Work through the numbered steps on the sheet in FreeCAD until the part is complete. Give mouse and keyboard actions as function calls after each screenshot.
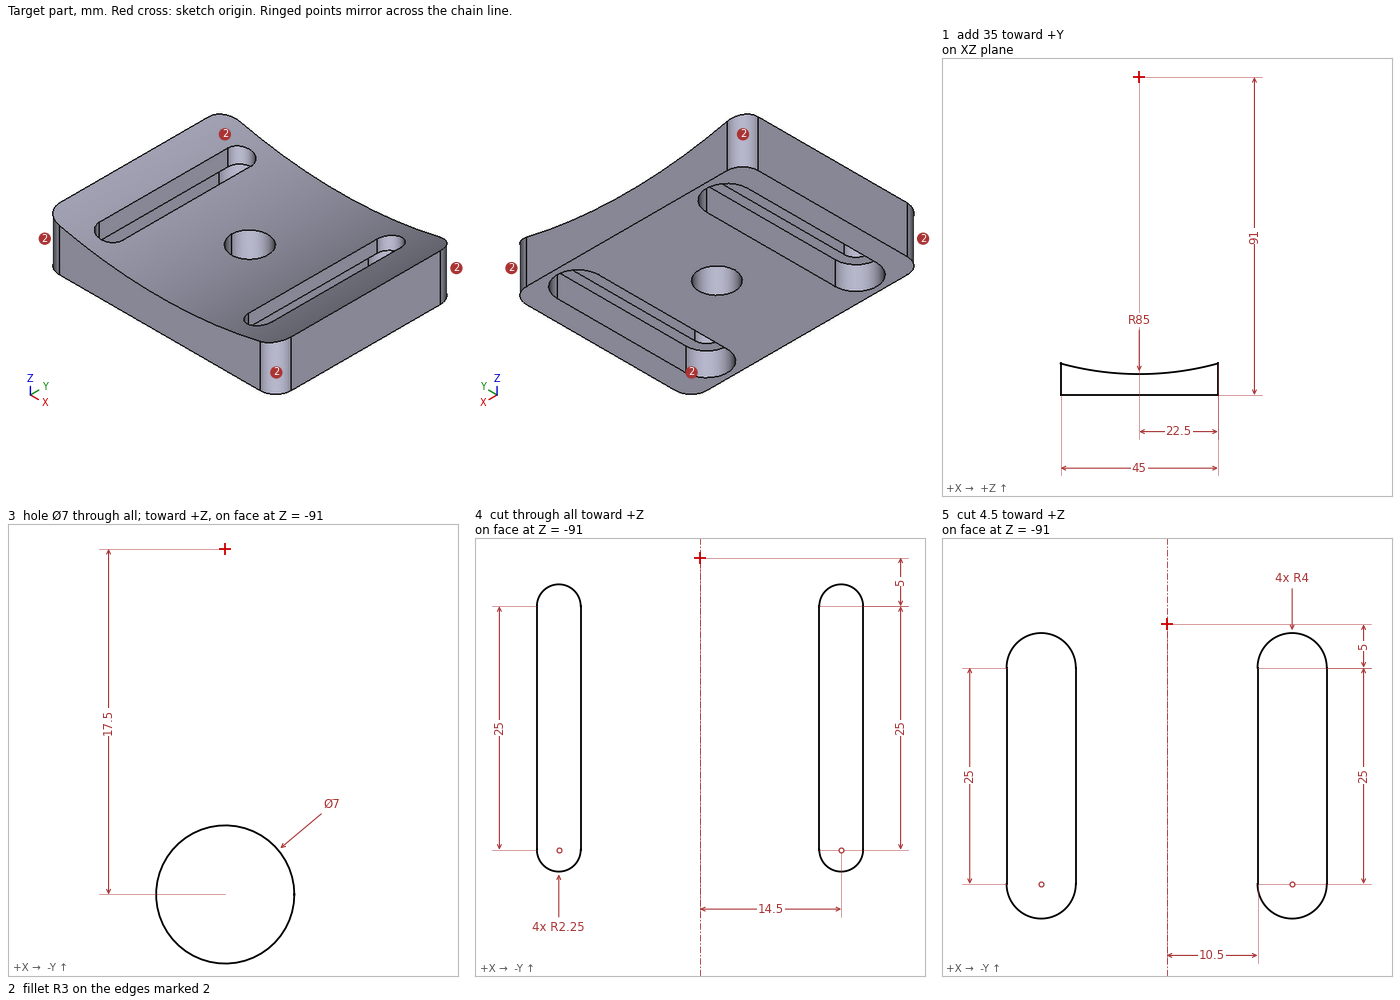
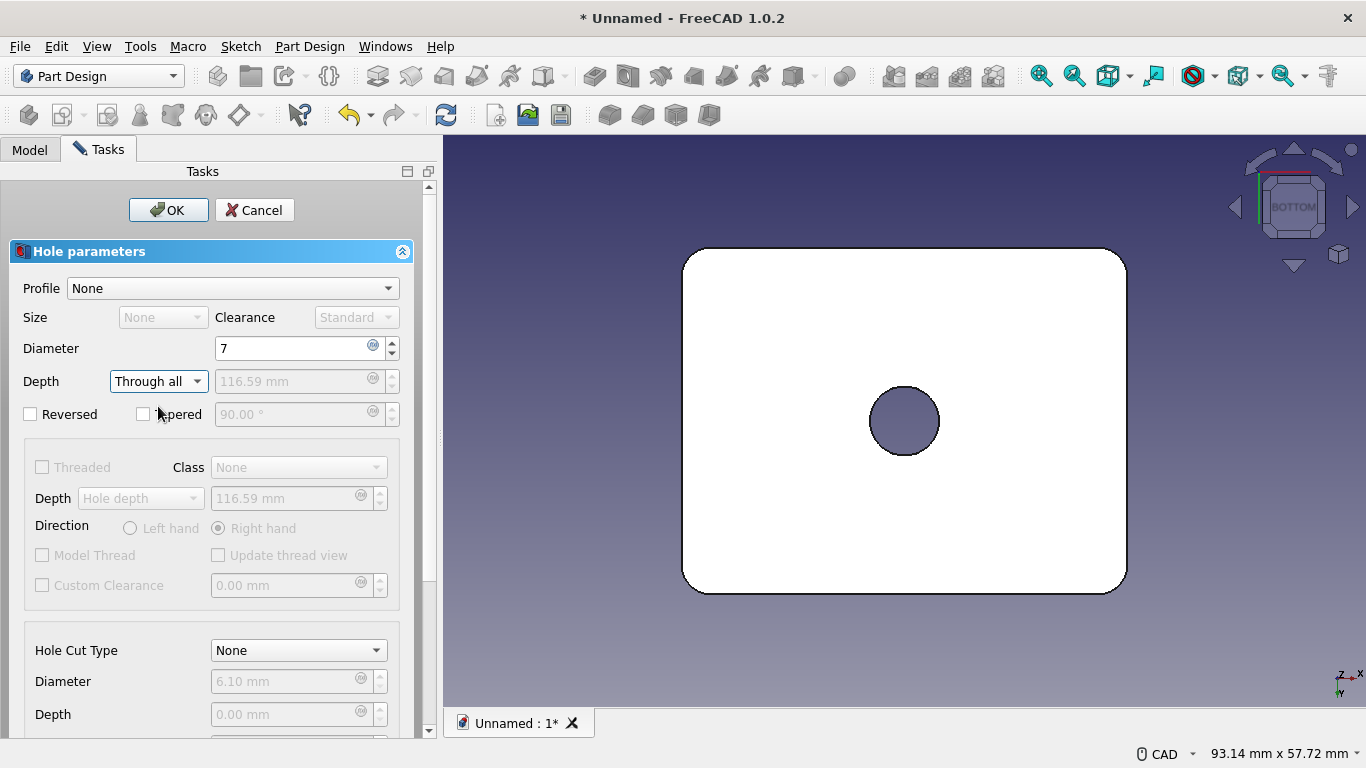
click(169, 210)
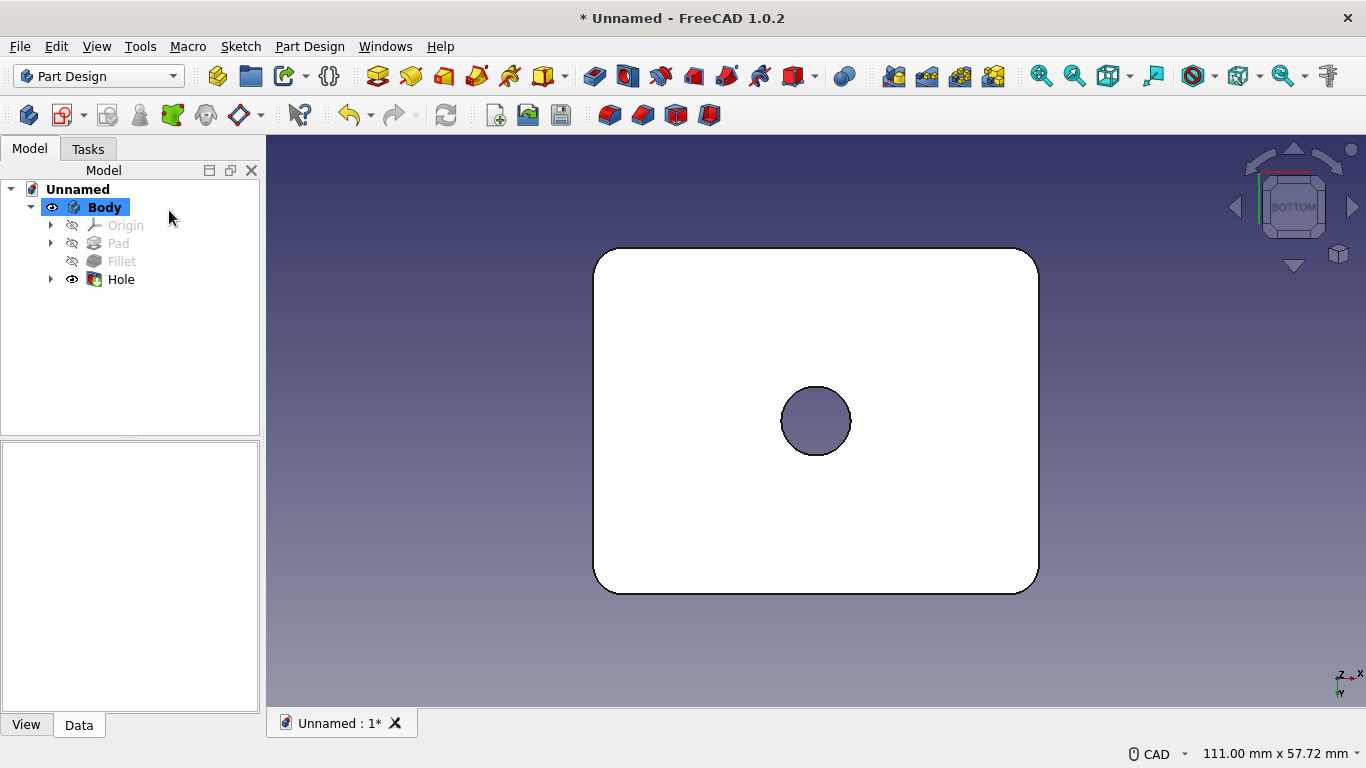
click(943, 470)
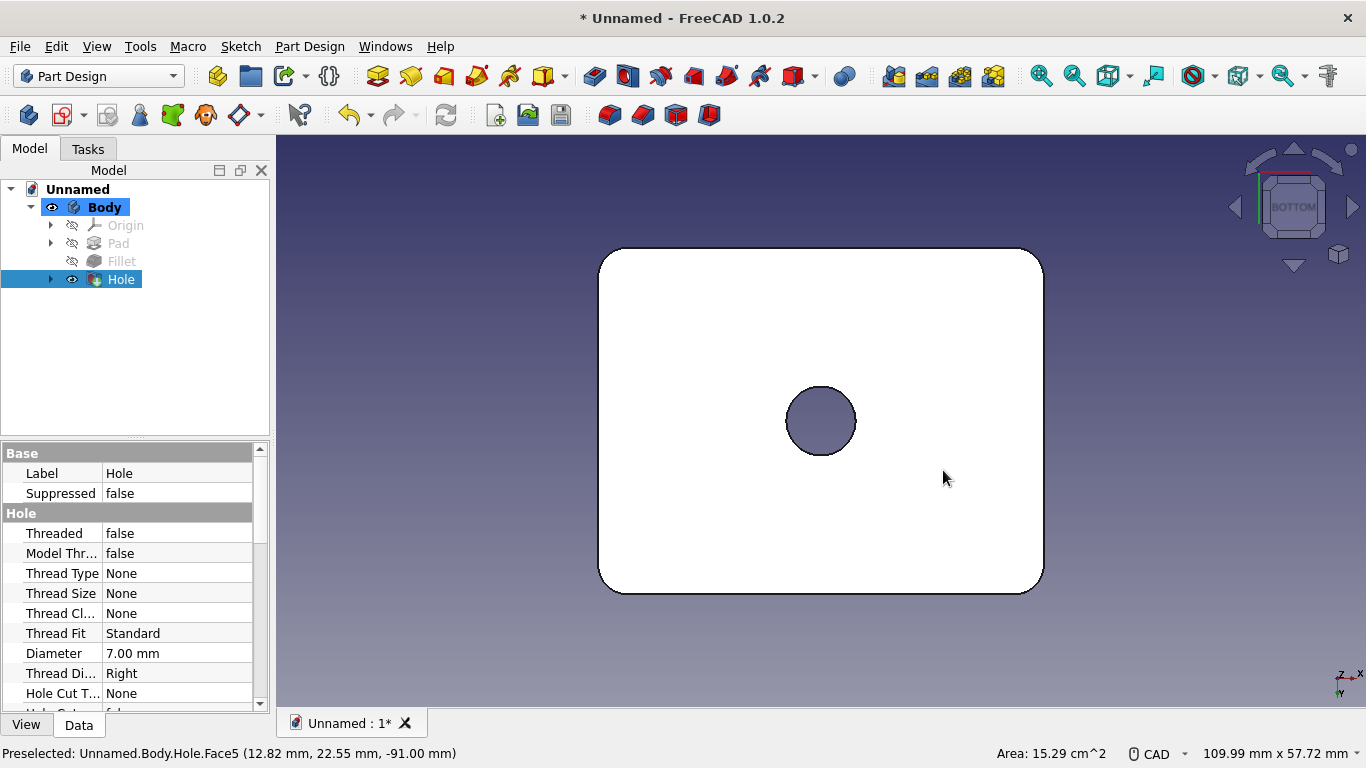
click(62, 116)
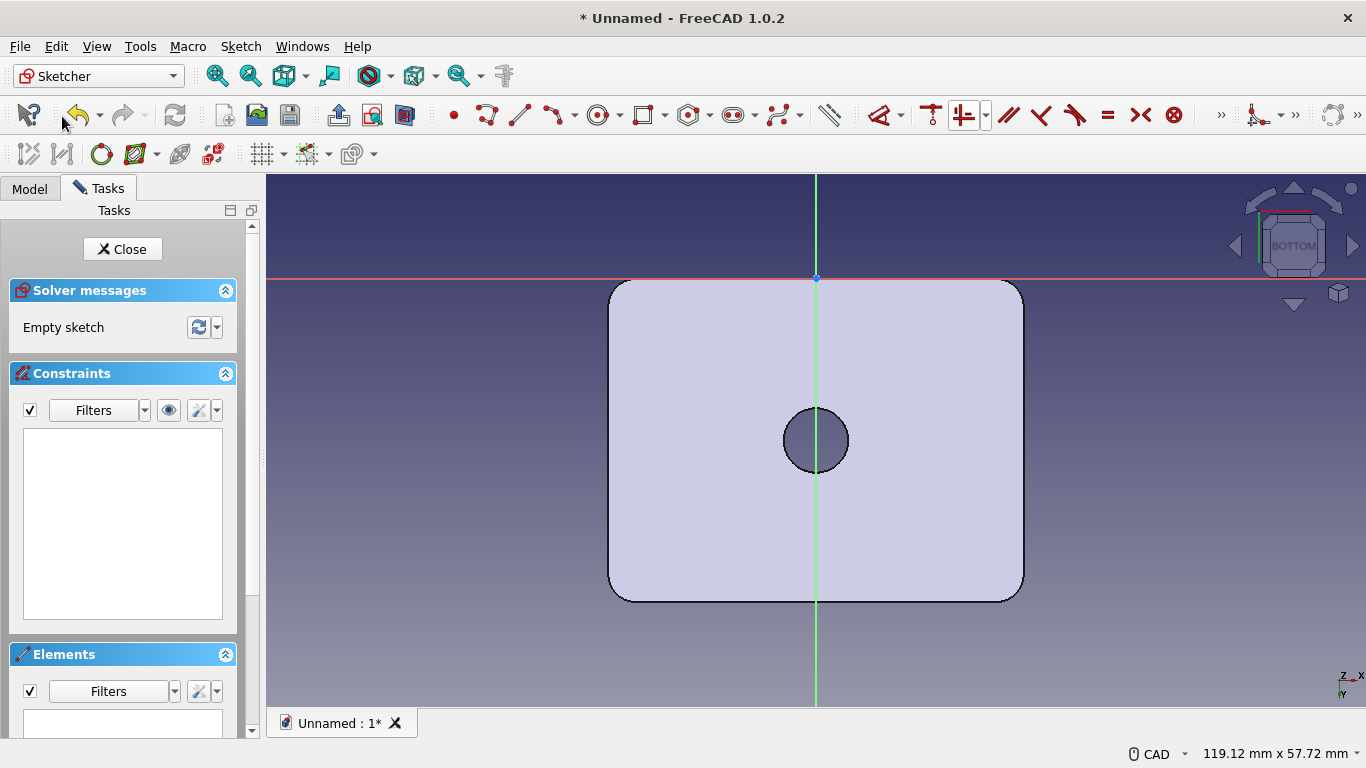
key(g)
key(s)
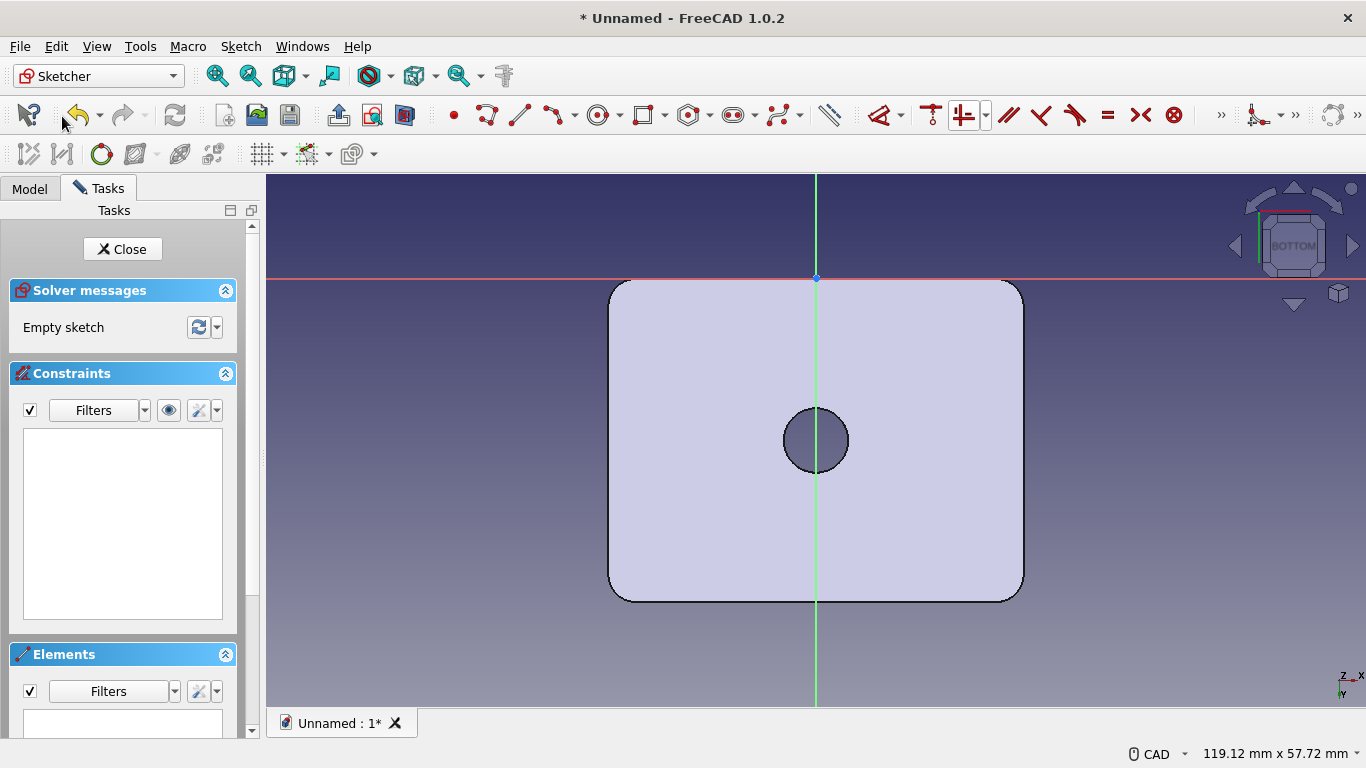
click(950, 556)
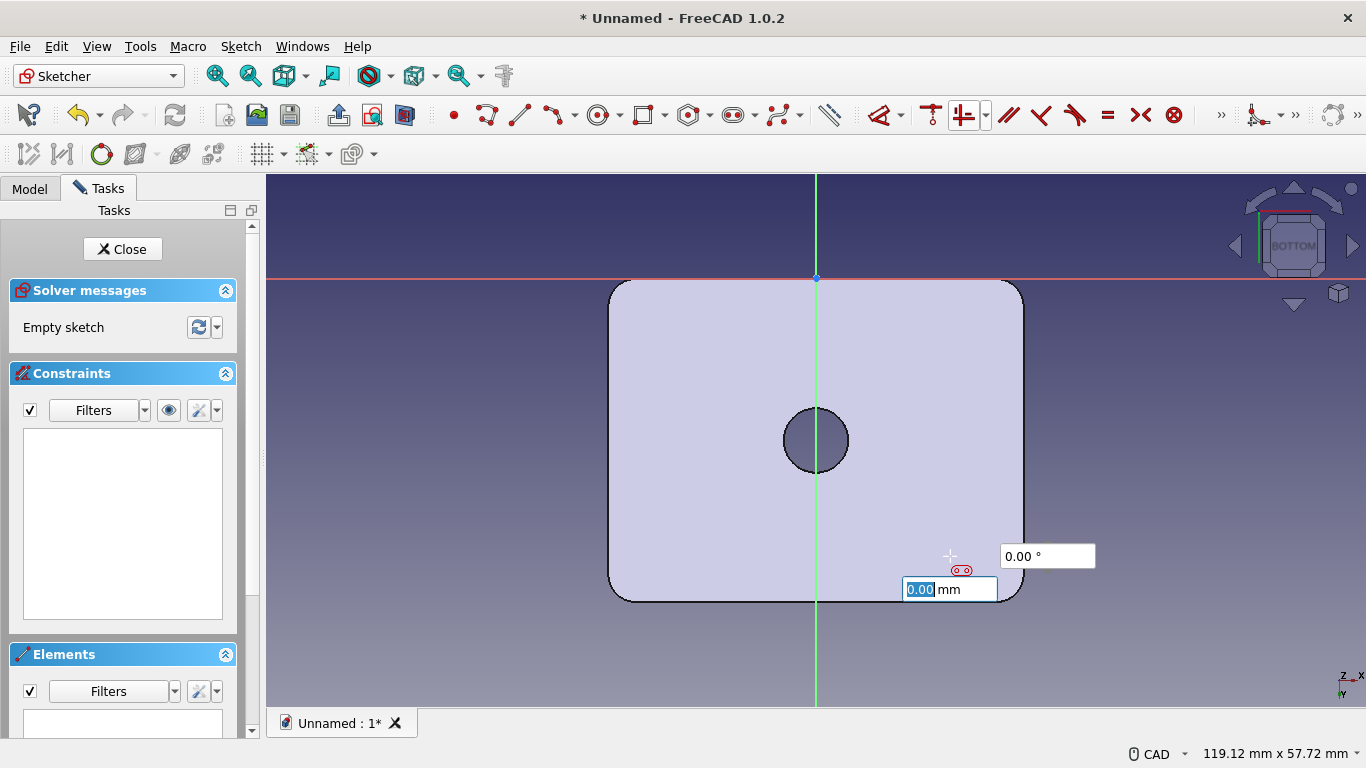
click(950, 325)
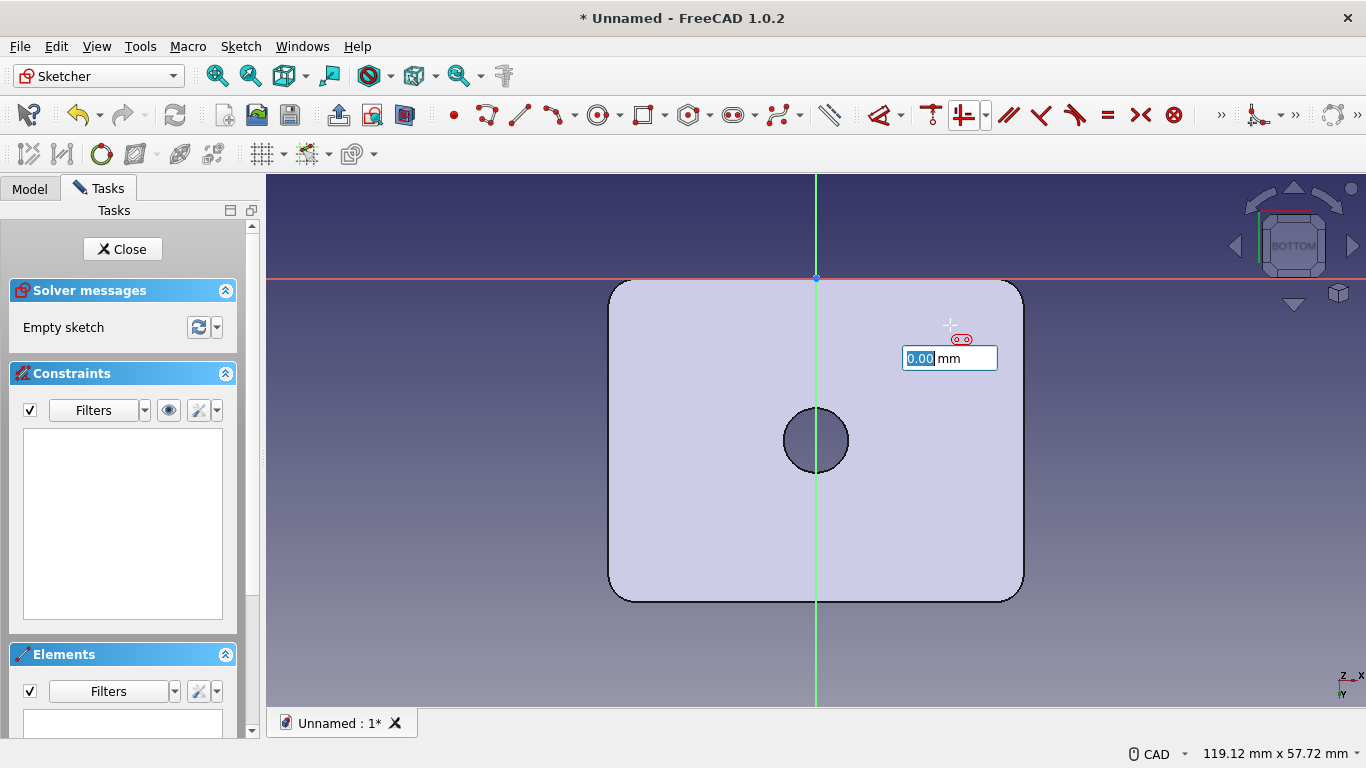
click(929, 440)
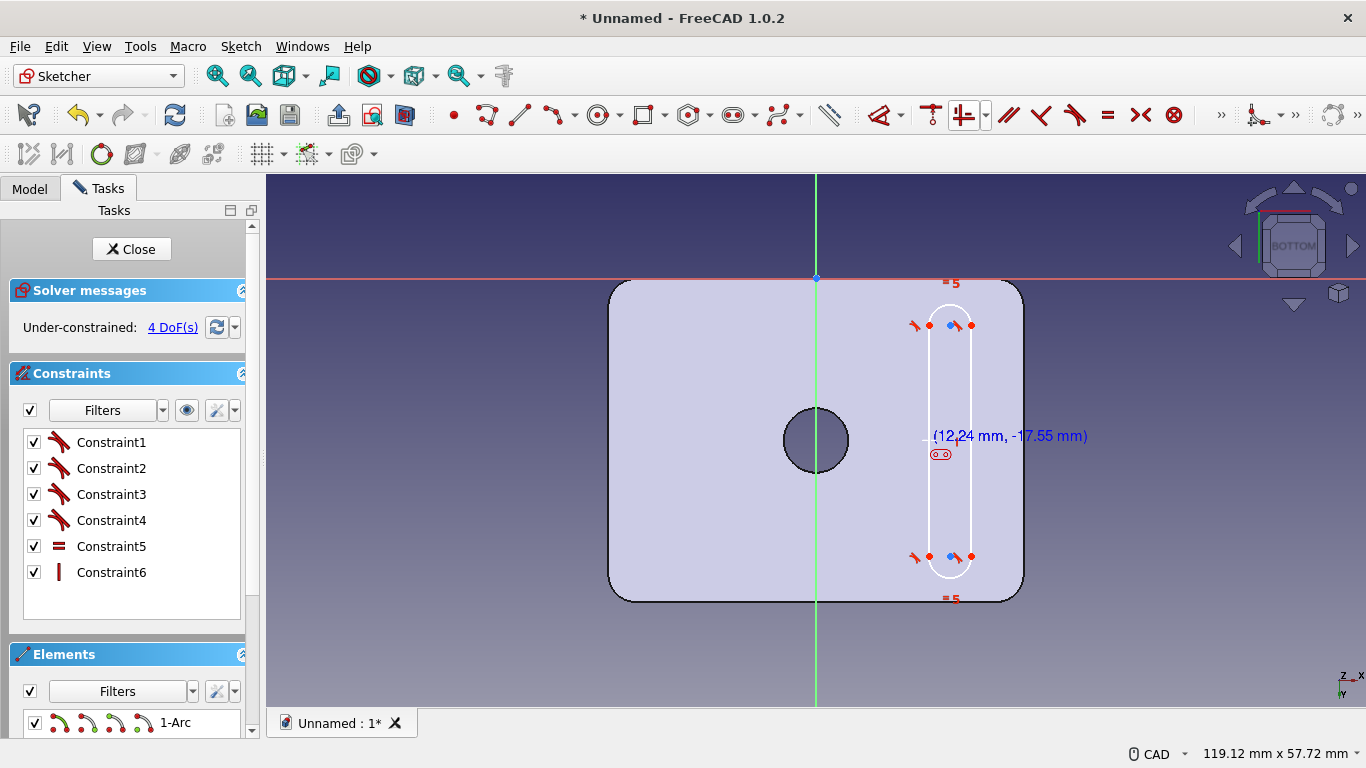
click(682, 556)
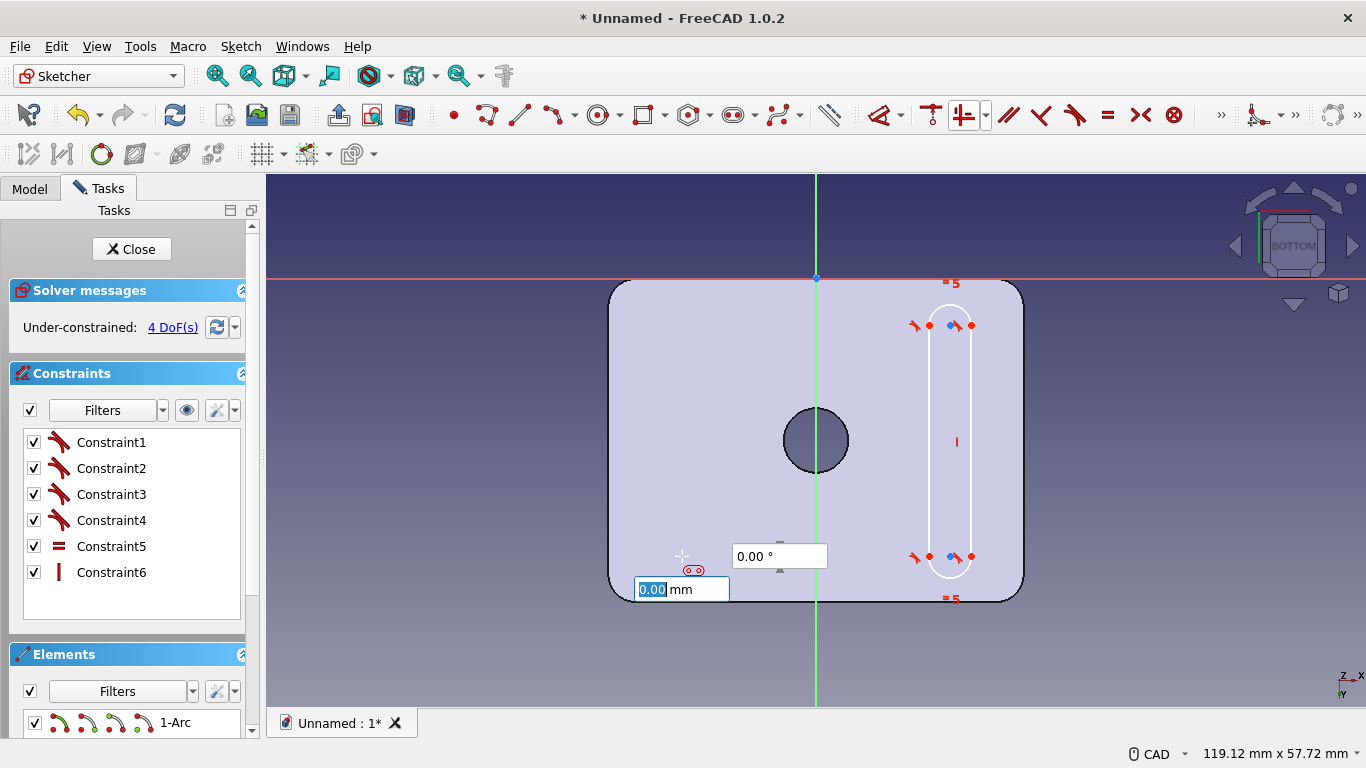
click(682, 325)